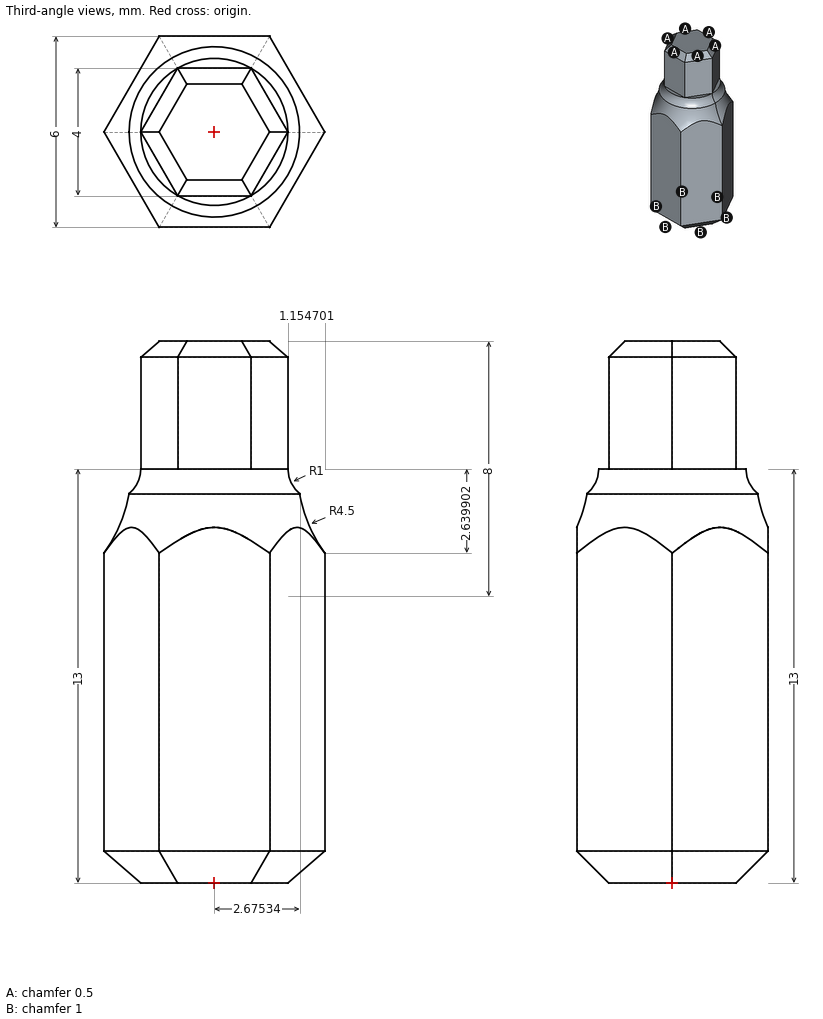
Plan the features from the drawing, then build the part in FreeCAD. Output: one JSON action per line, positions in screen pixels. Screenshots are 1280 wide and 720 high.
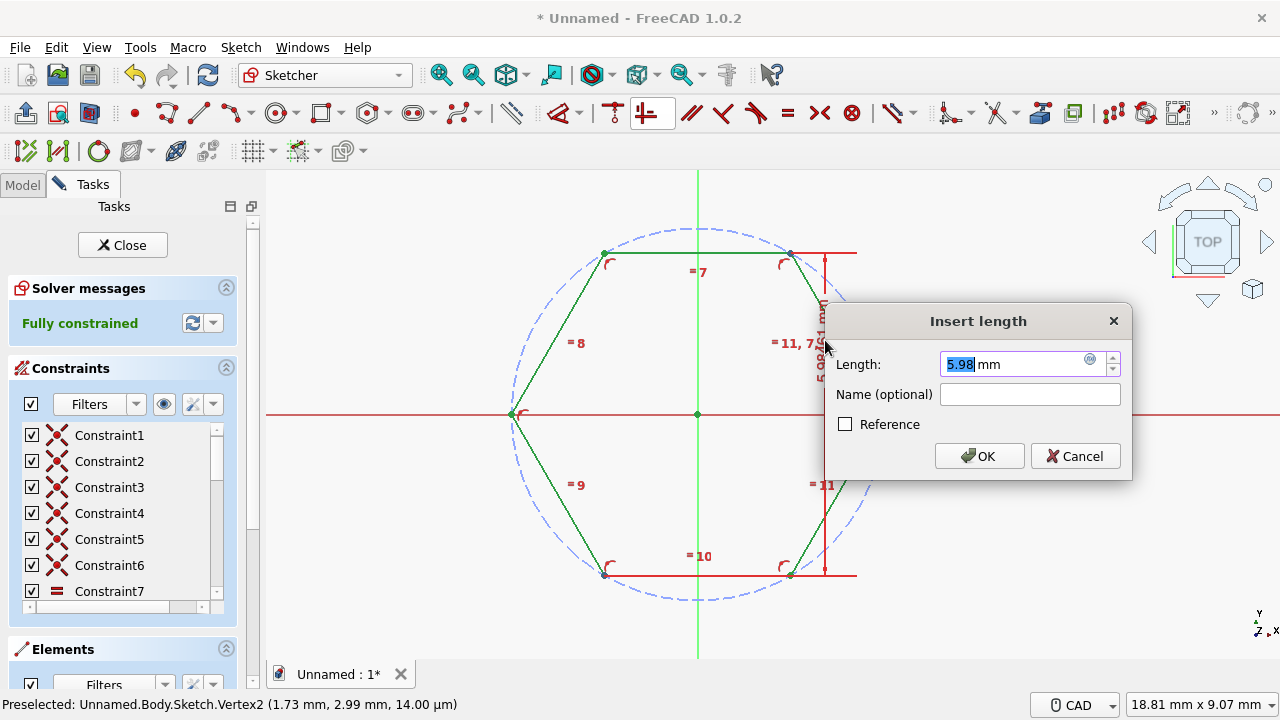
{"action": "type", "text": "6"}
{"action": "key", "text": "Return"}
{"action": "key", "text": "Escape"}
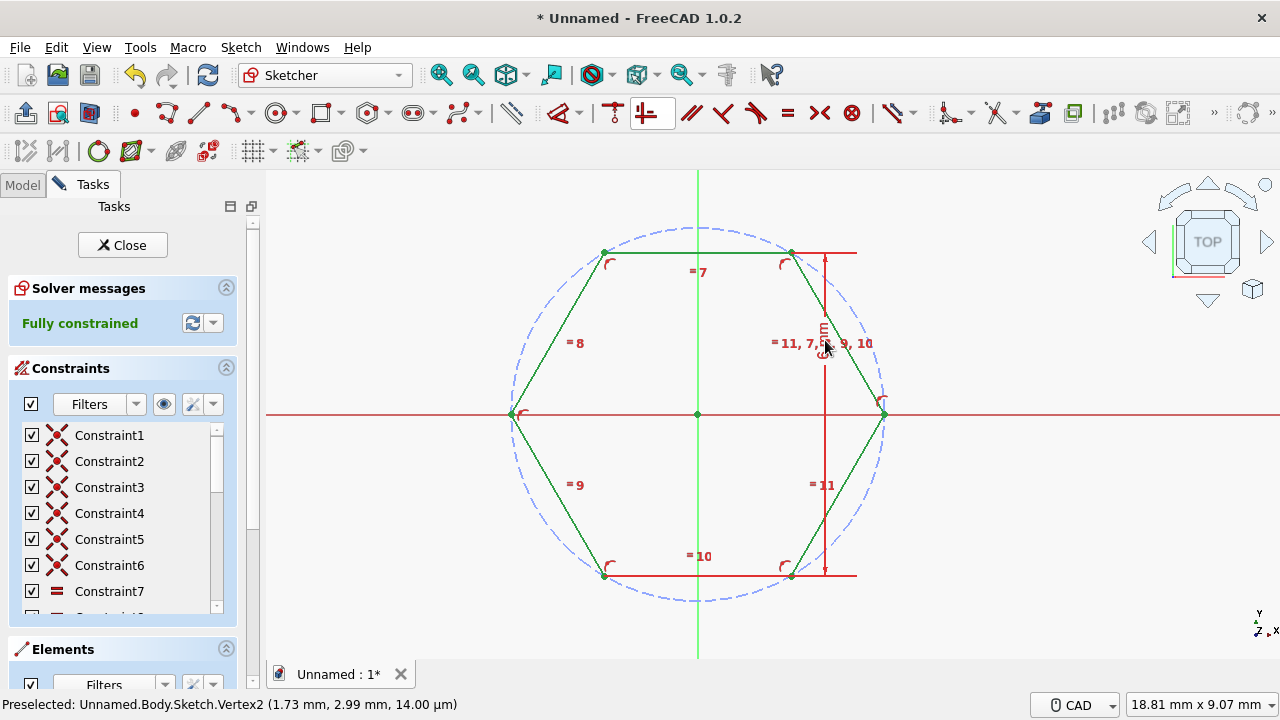
{"action": "left_click", "coordinate": [123, 245]}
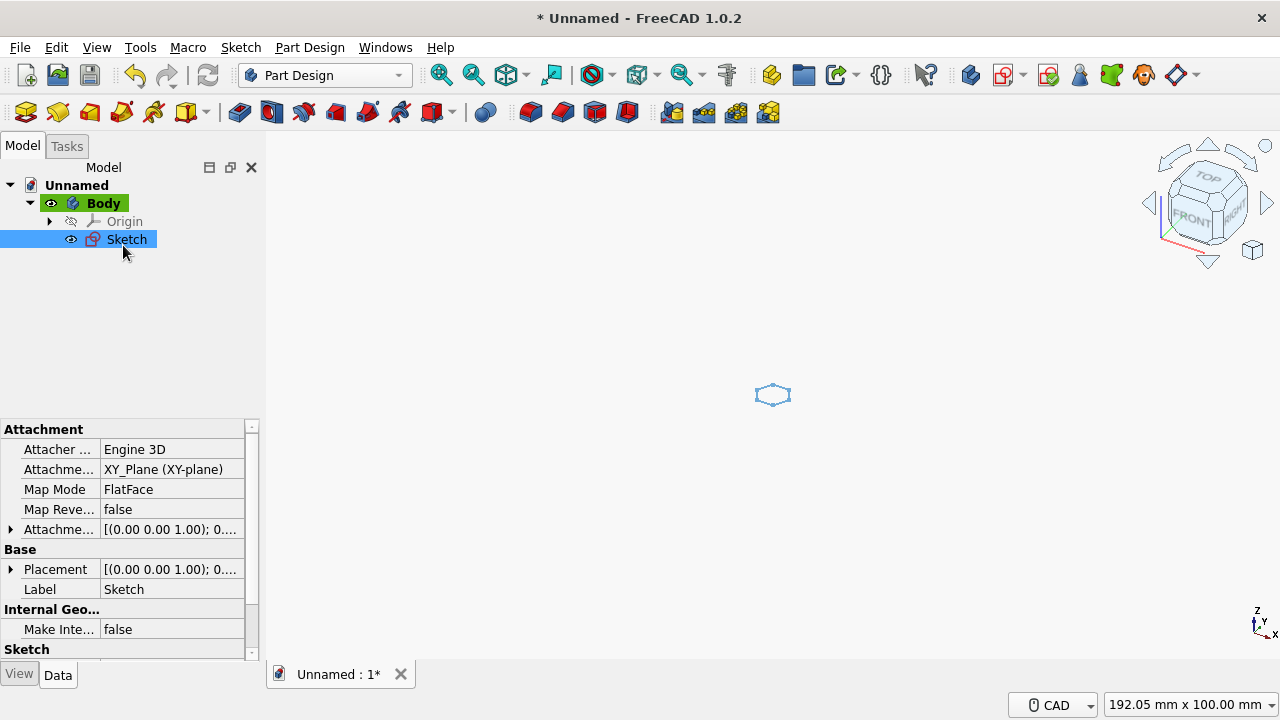
{"action": "left_click", "coordinate": [26, 112]}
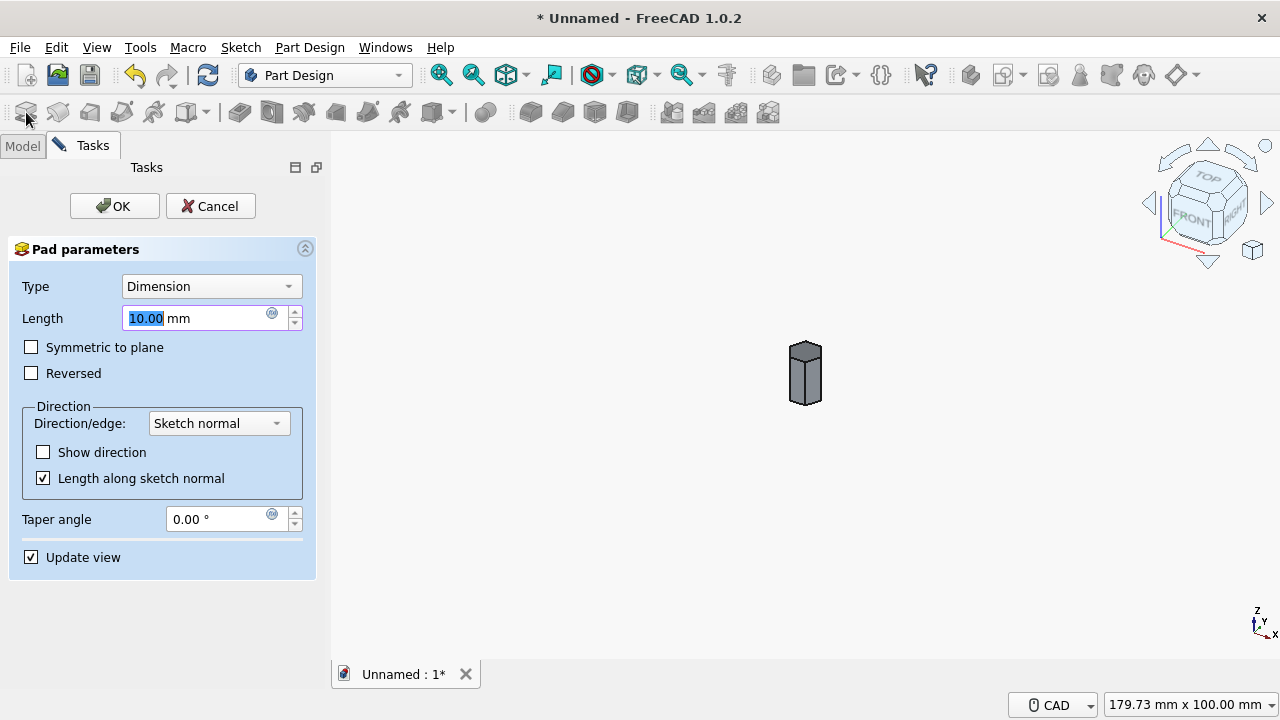
{"action": "type", "text": "13"}
{"action": "key", "text": "Tab"}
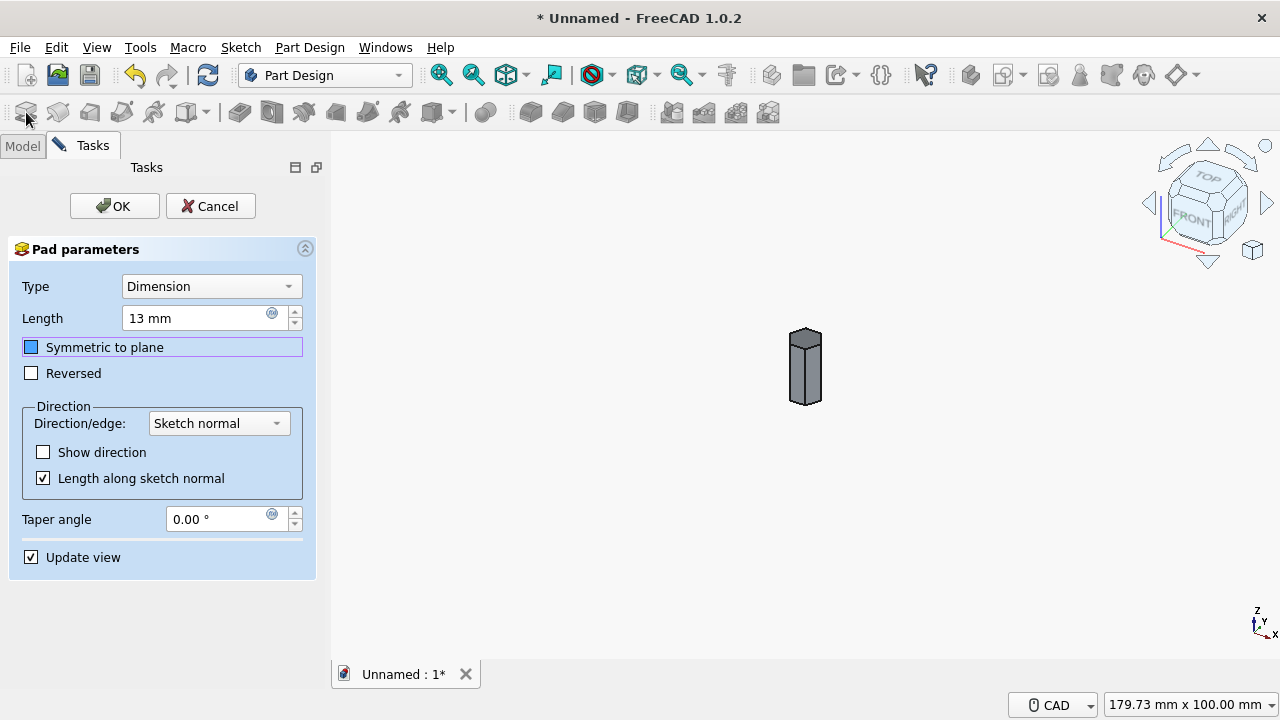
{"action": "left_click", "coordinate": [115, 206]}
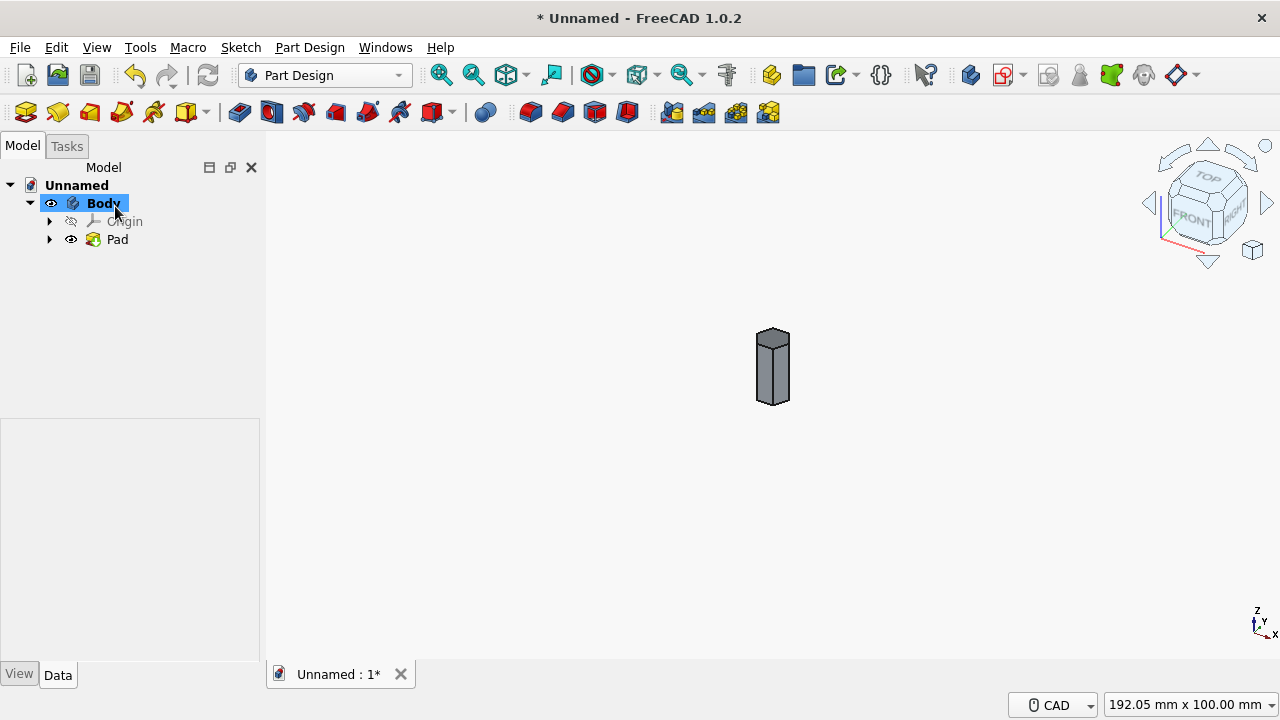
{"action": "left_click", "coordinate": [442, 76]}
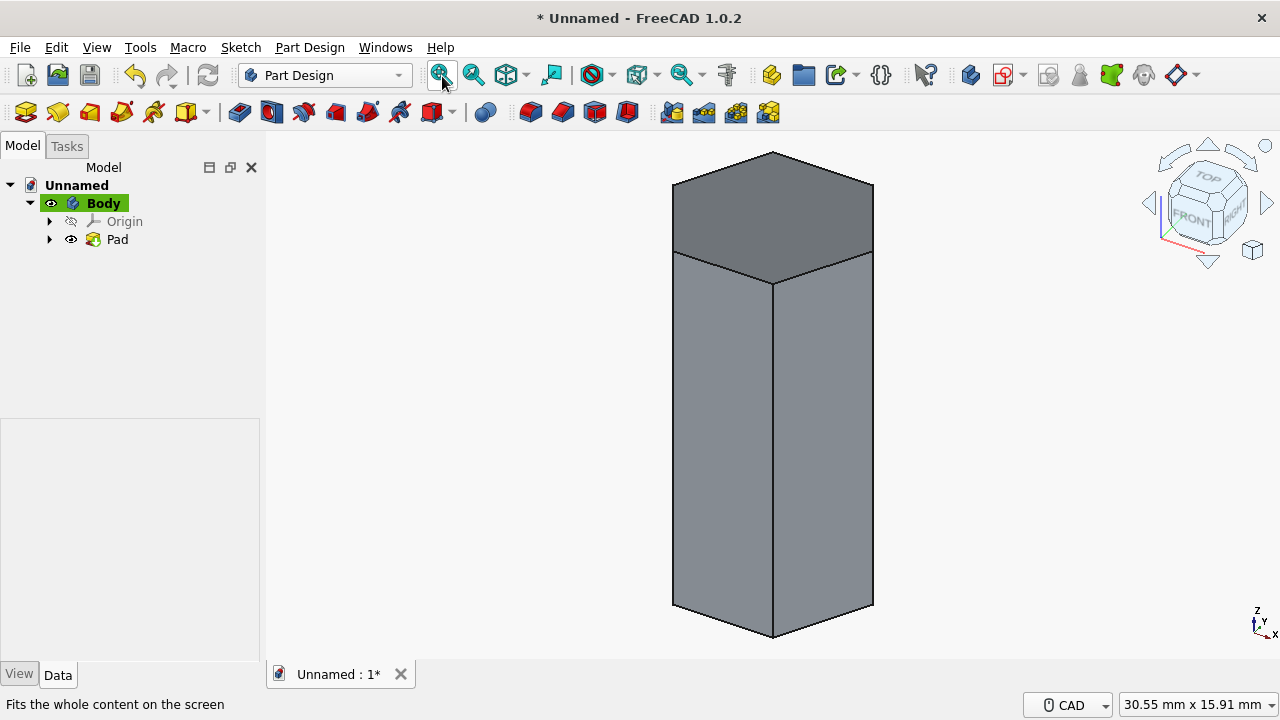
{"action": "left_click", "coordinate": [773, 217]}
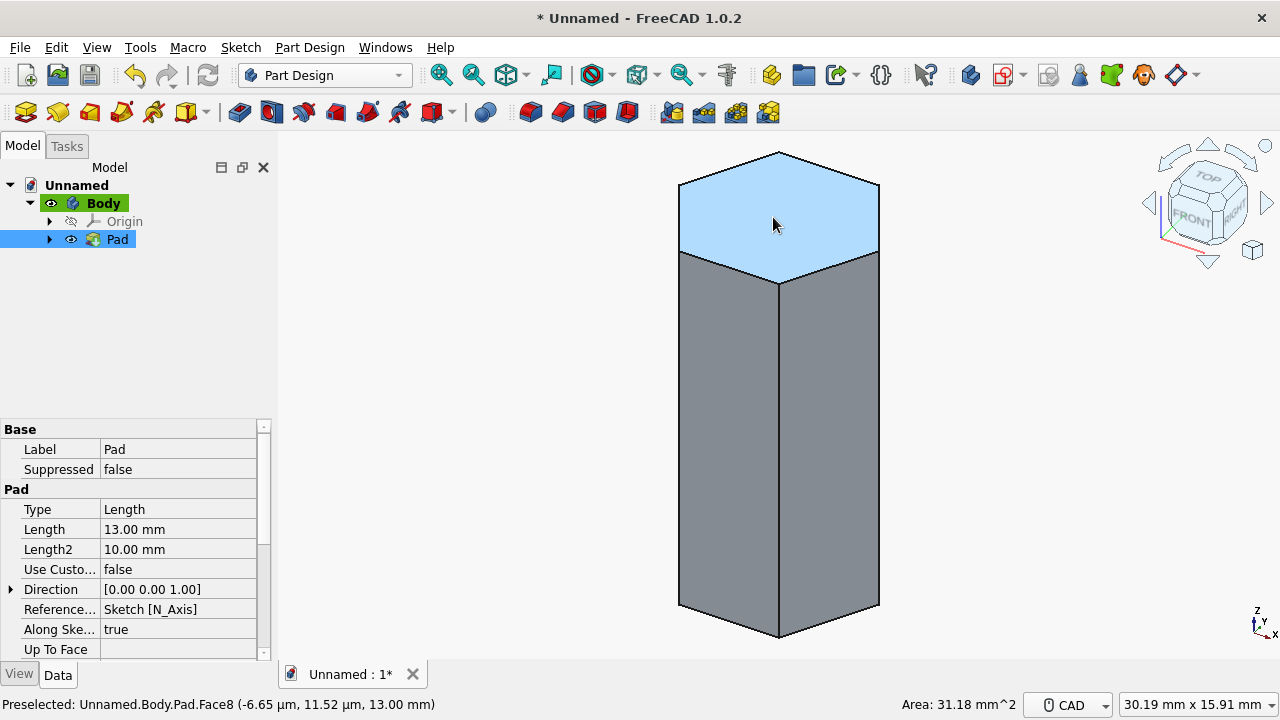
{"action": "left_click", "coordinate": [1004, 76]}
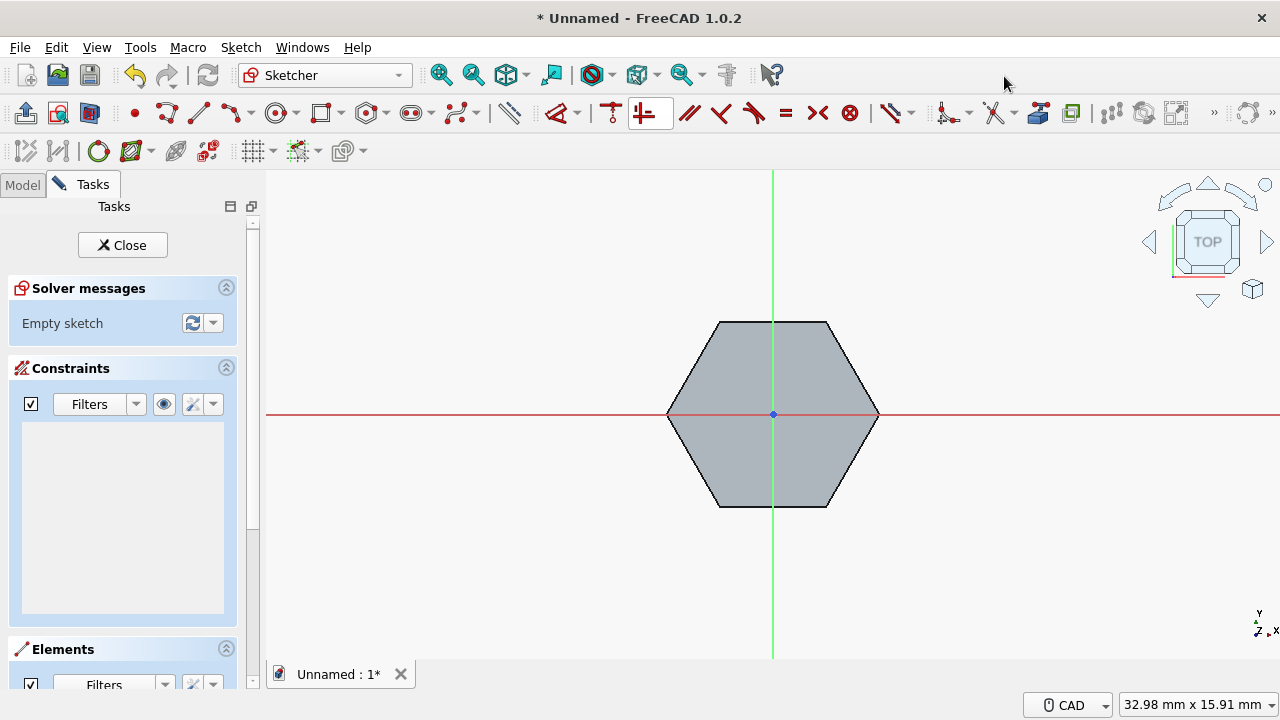
{"action": "scroll", "coordinate": [813, 415], "scroll_direction": "up", "scroll_amount": 5}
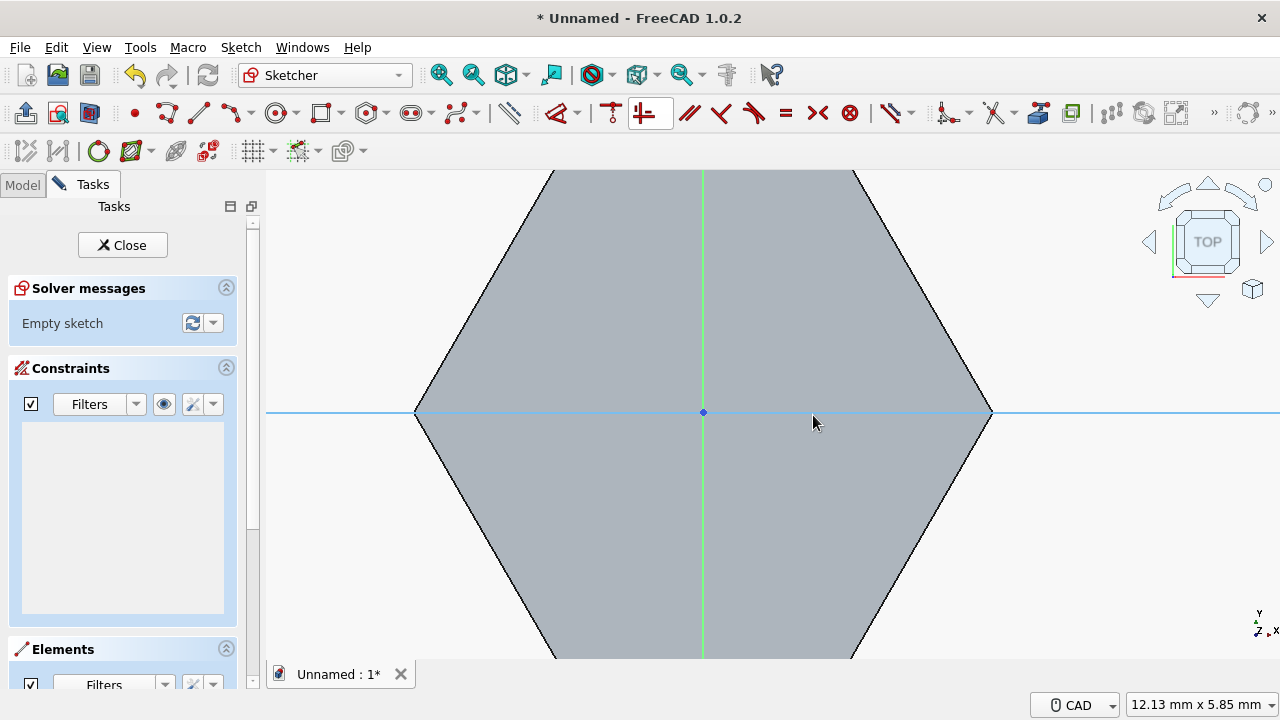
{"action": "left_click", "coordinate": [366, 114]}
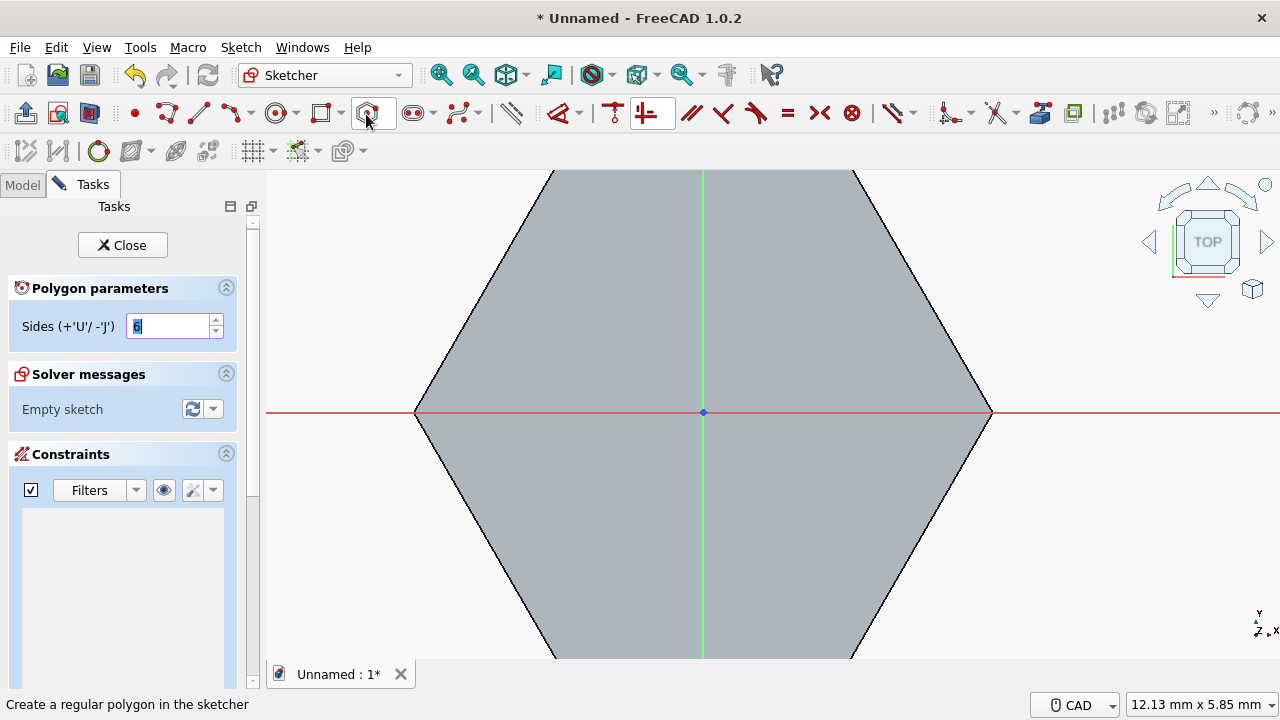
{"action": "left_click", "coordinate": [703, 413]}